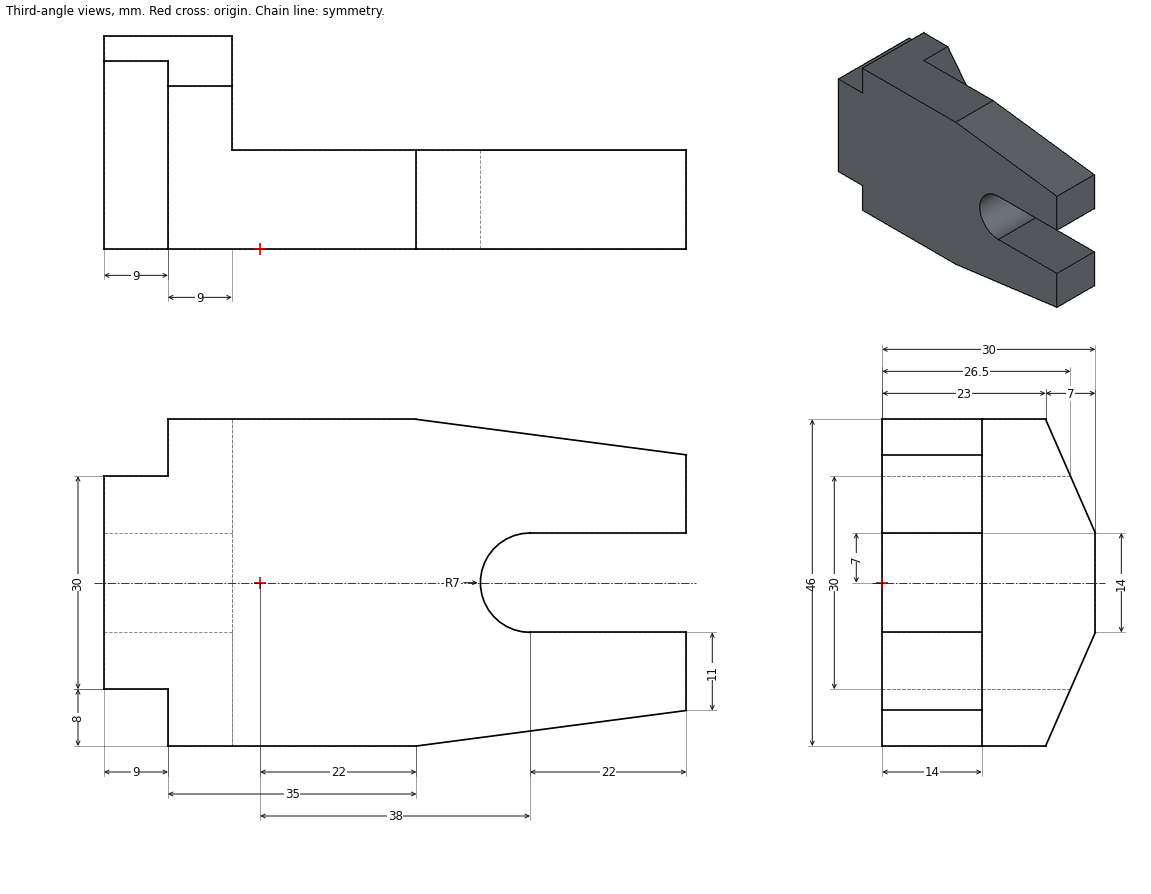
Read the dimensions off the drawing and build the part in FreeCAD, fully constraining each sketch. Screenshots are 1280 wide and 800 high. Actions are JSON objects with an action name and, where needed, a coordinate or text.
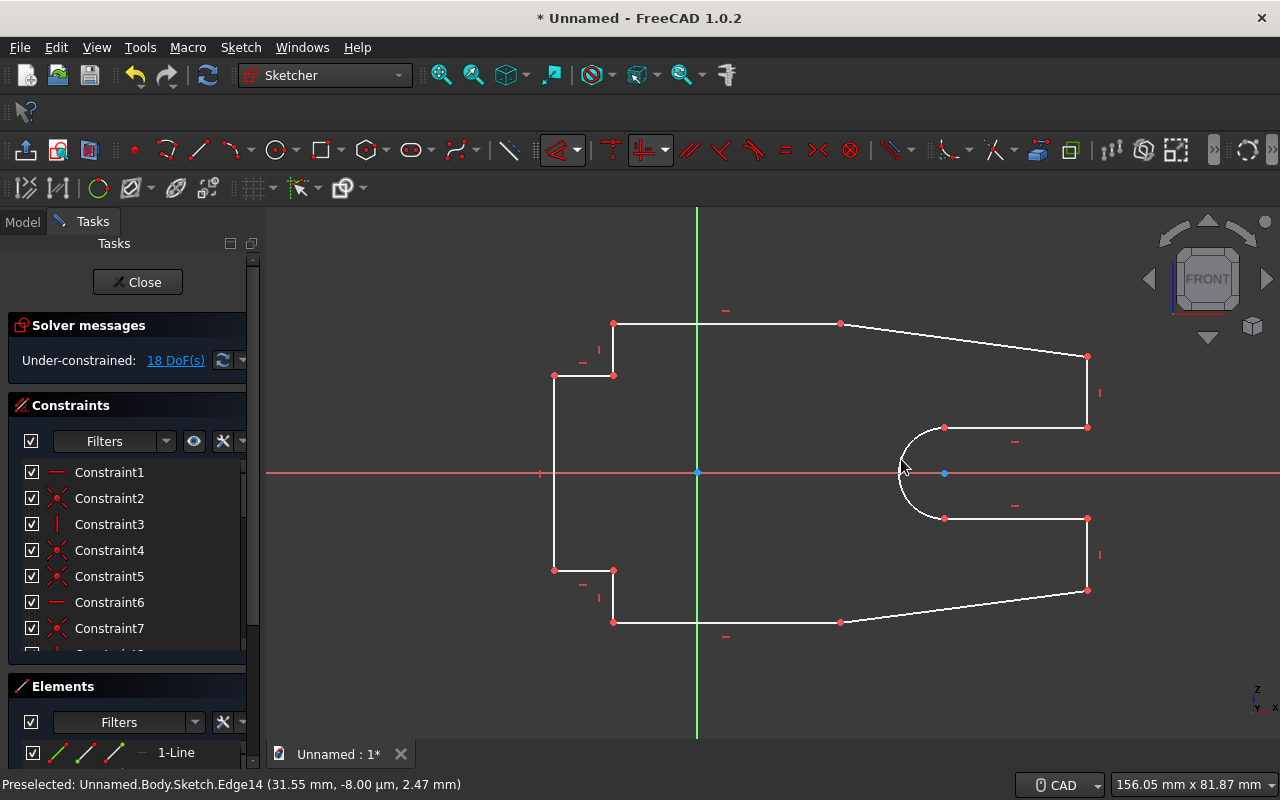
{"action": "left_click", "coordinate": [987, 519]}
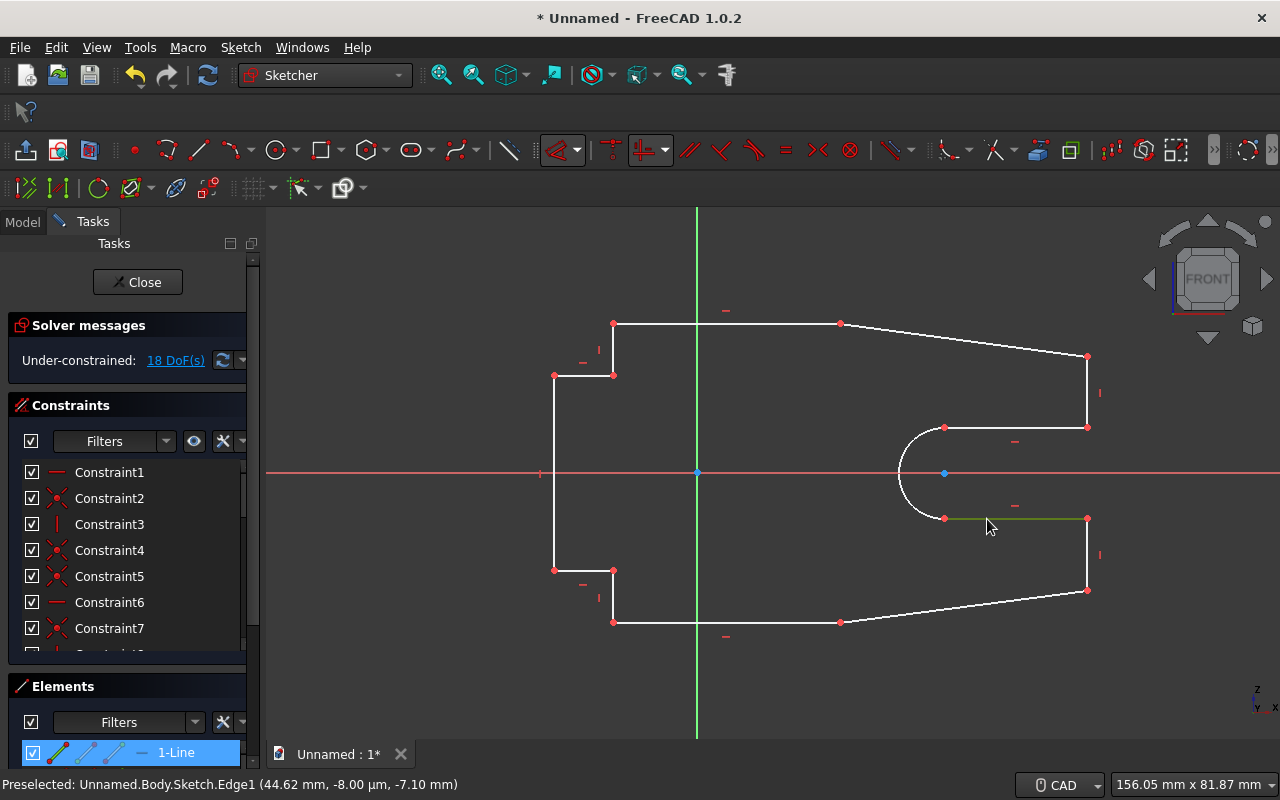
{"action": "left_click", "coordinate": [908, 447]}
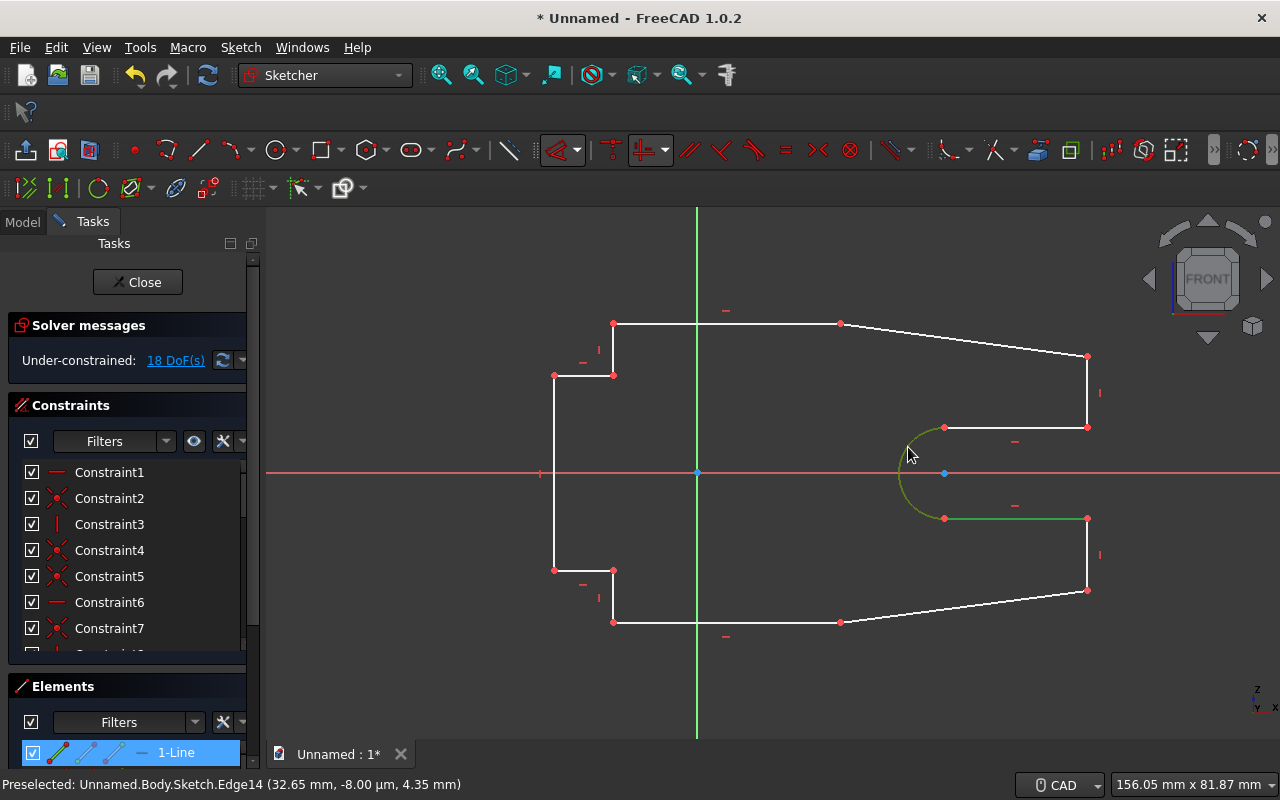
{"action": "left_click", "coordinate": [754, 150]}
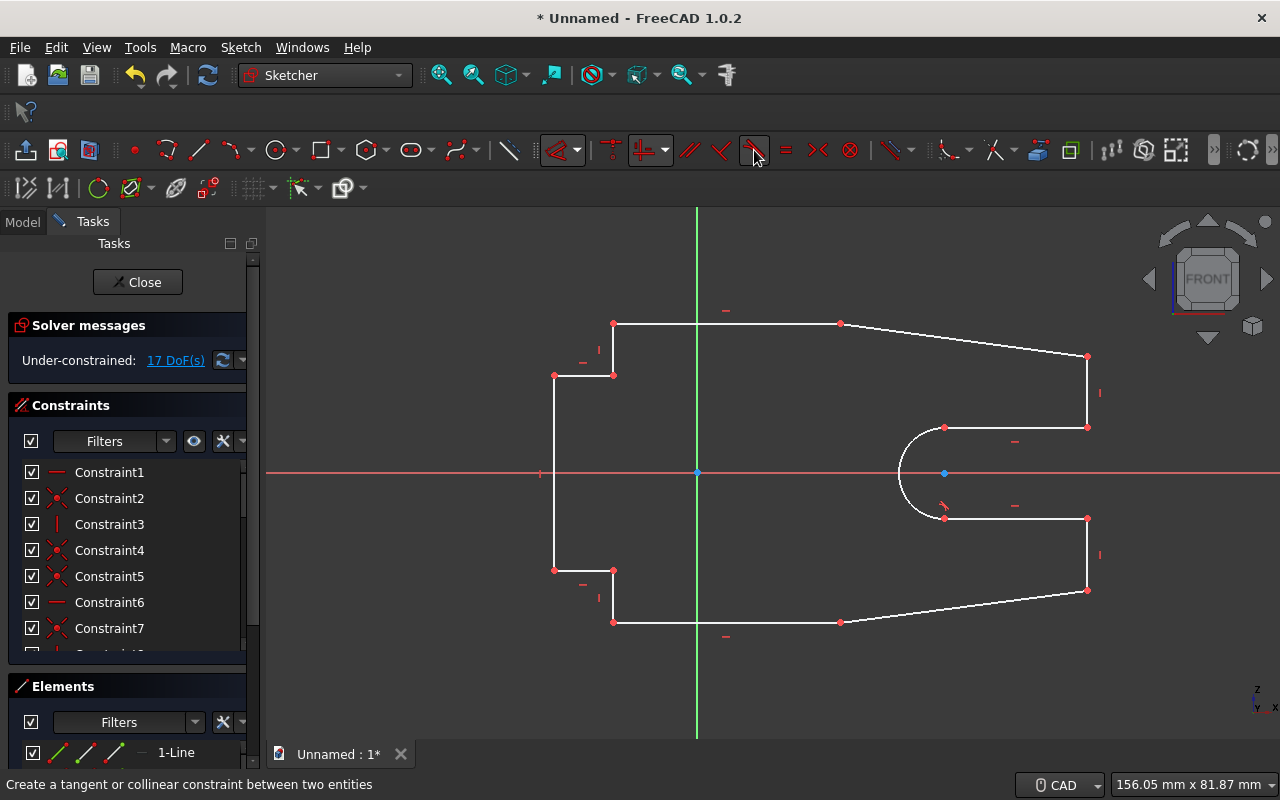
{"action": "left_click", "coordinate": [1044, 428]}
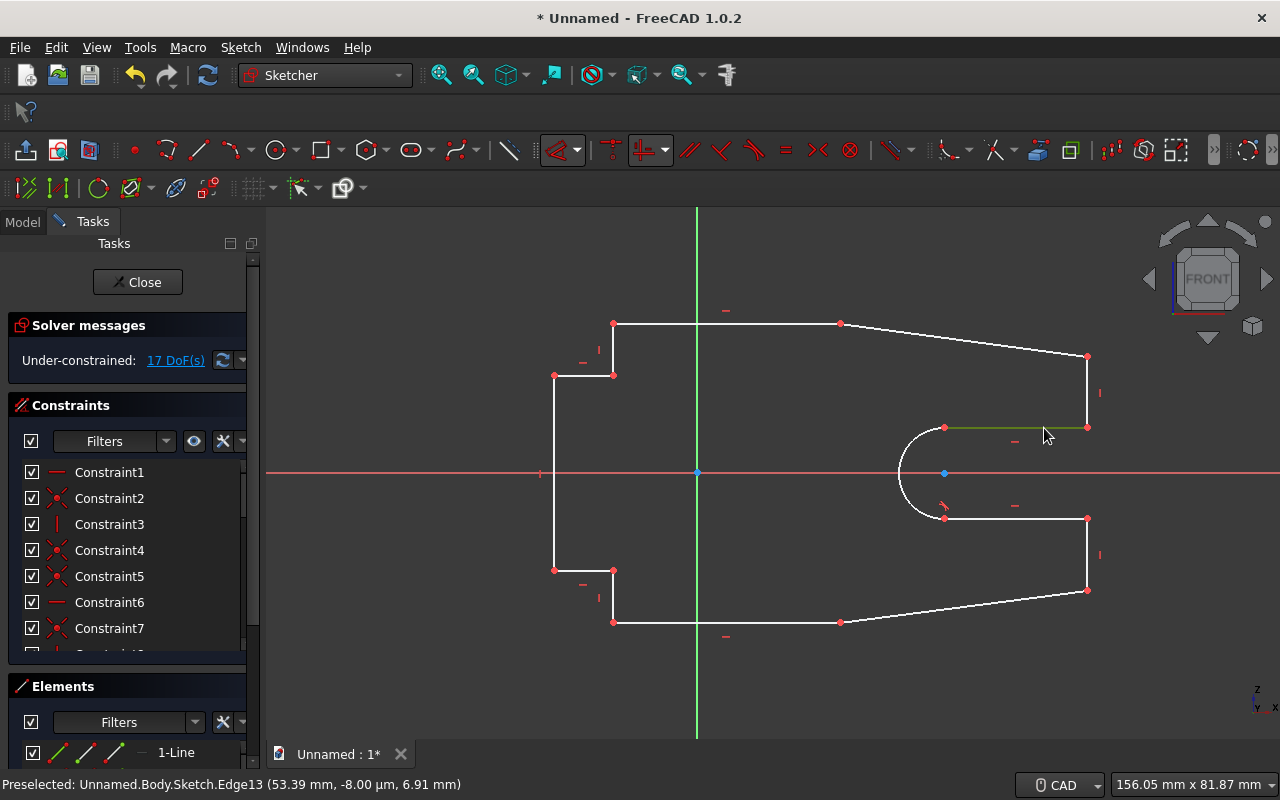
{"action": "left_click", "coordinate": [907, 447]}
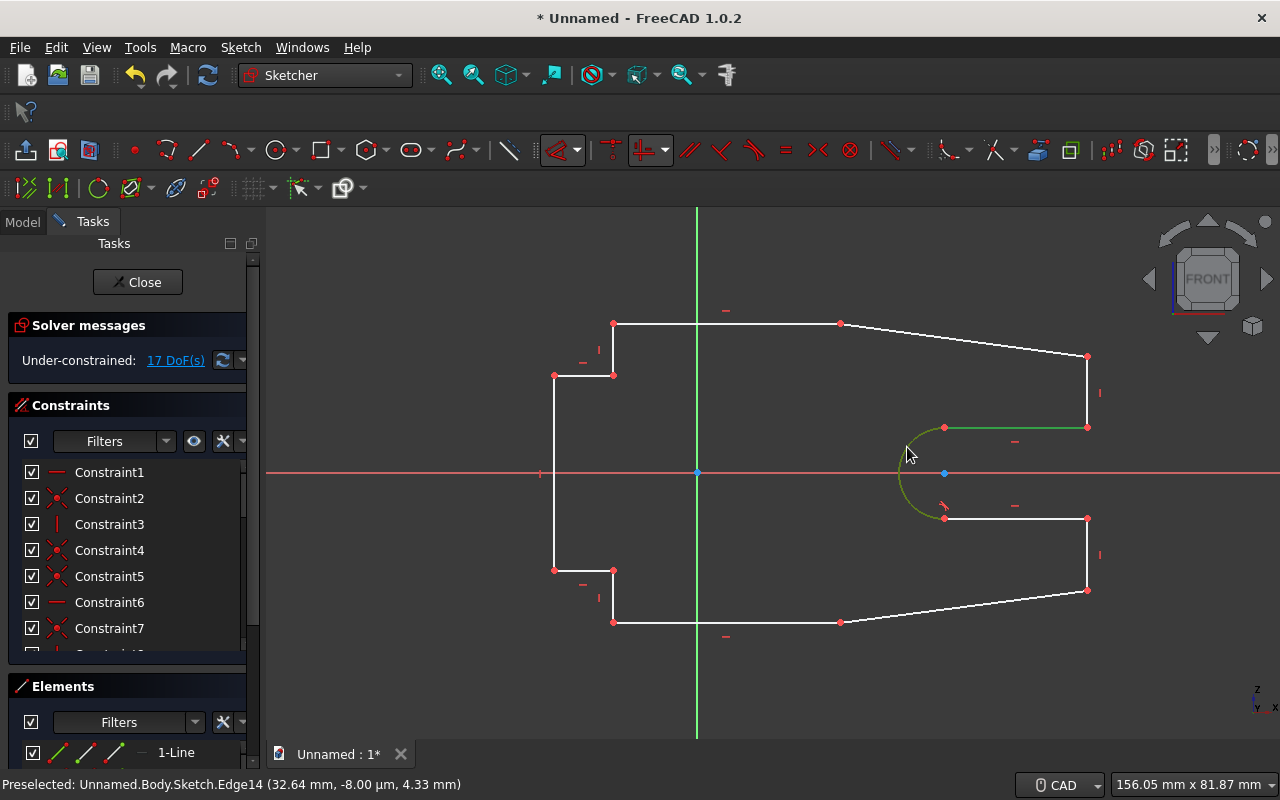
{"action": "key", "text": "t"}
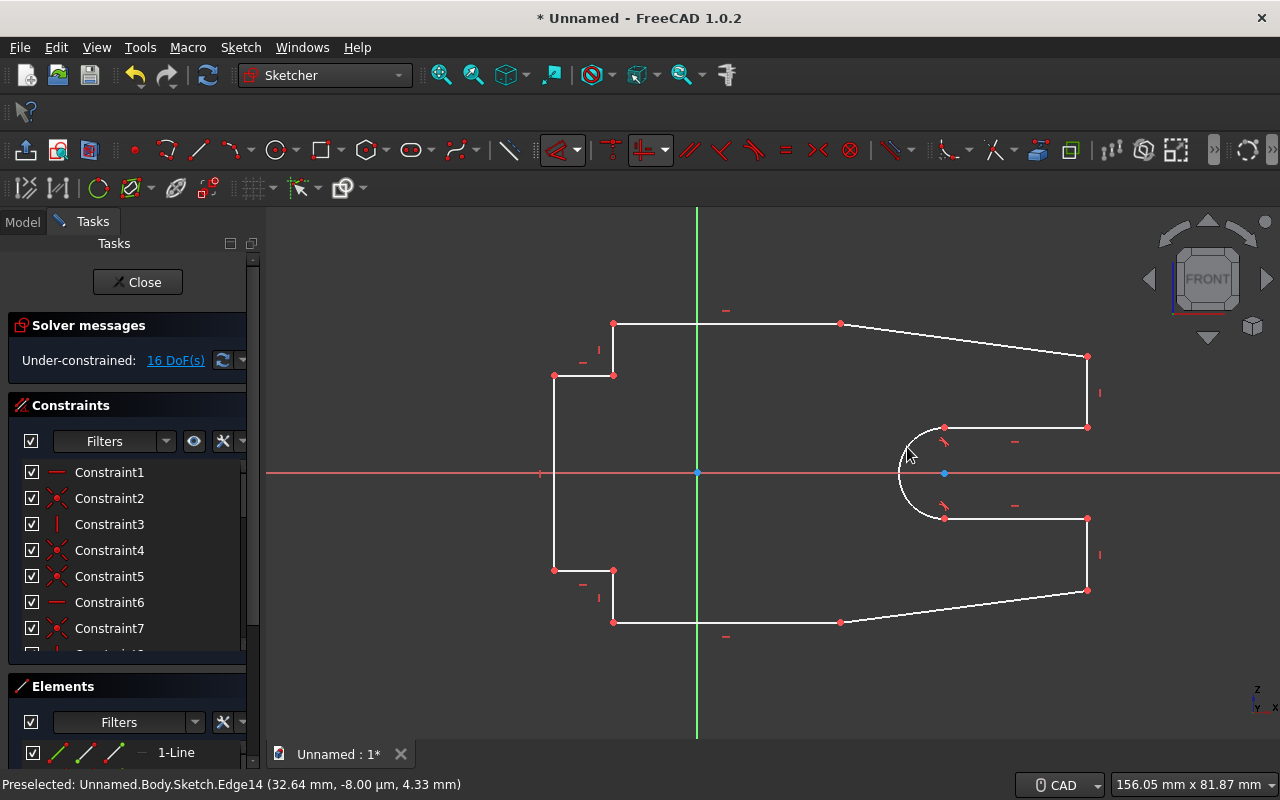
{"action": "left_click", "coordinate": [944, 474]}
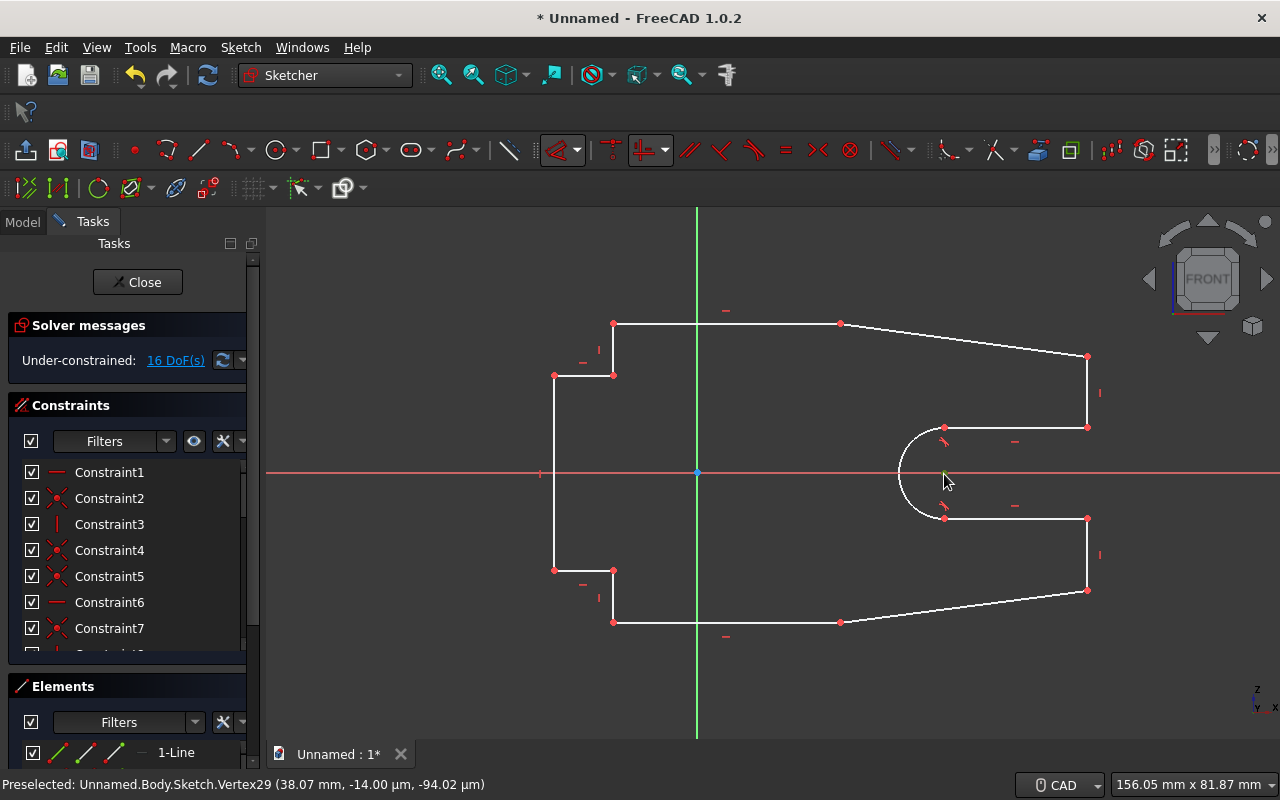
{"action": "left_click", "coordinate": [353, 473]}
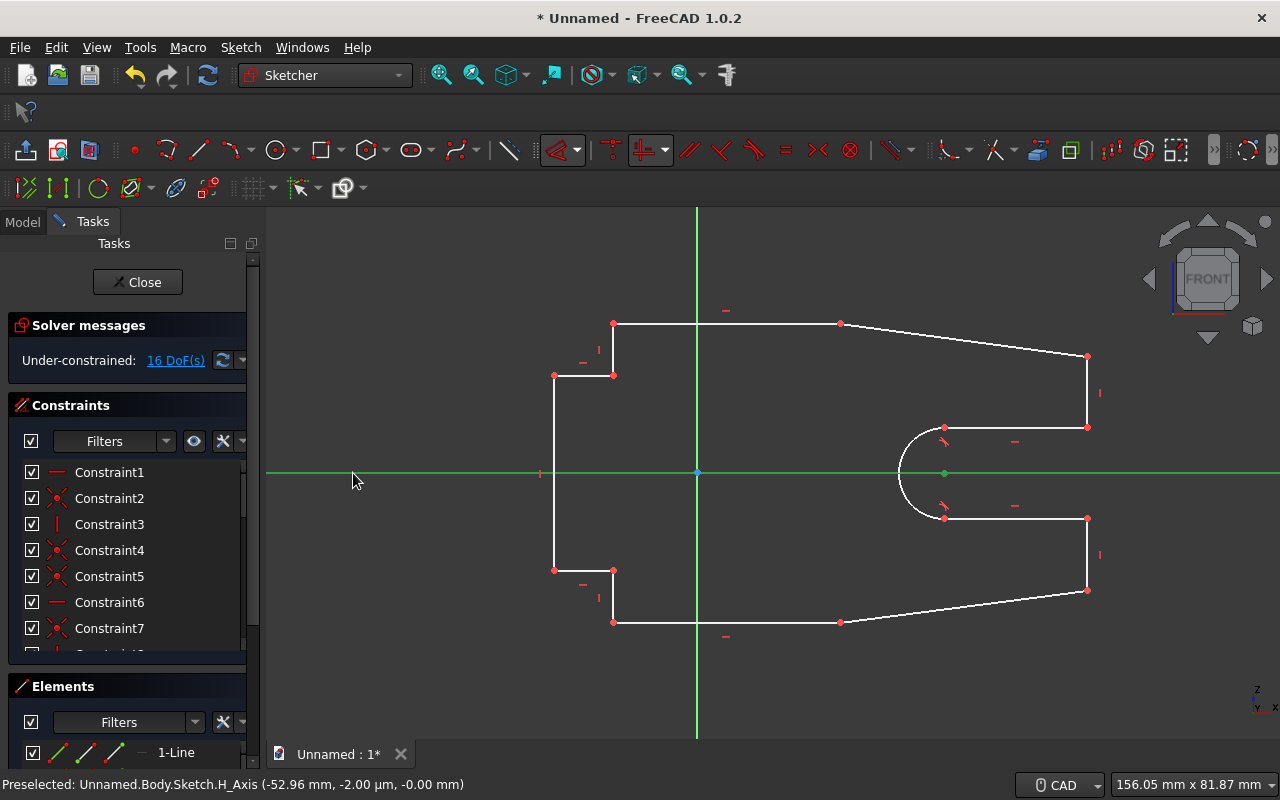
{"action": "key", "text": "c"}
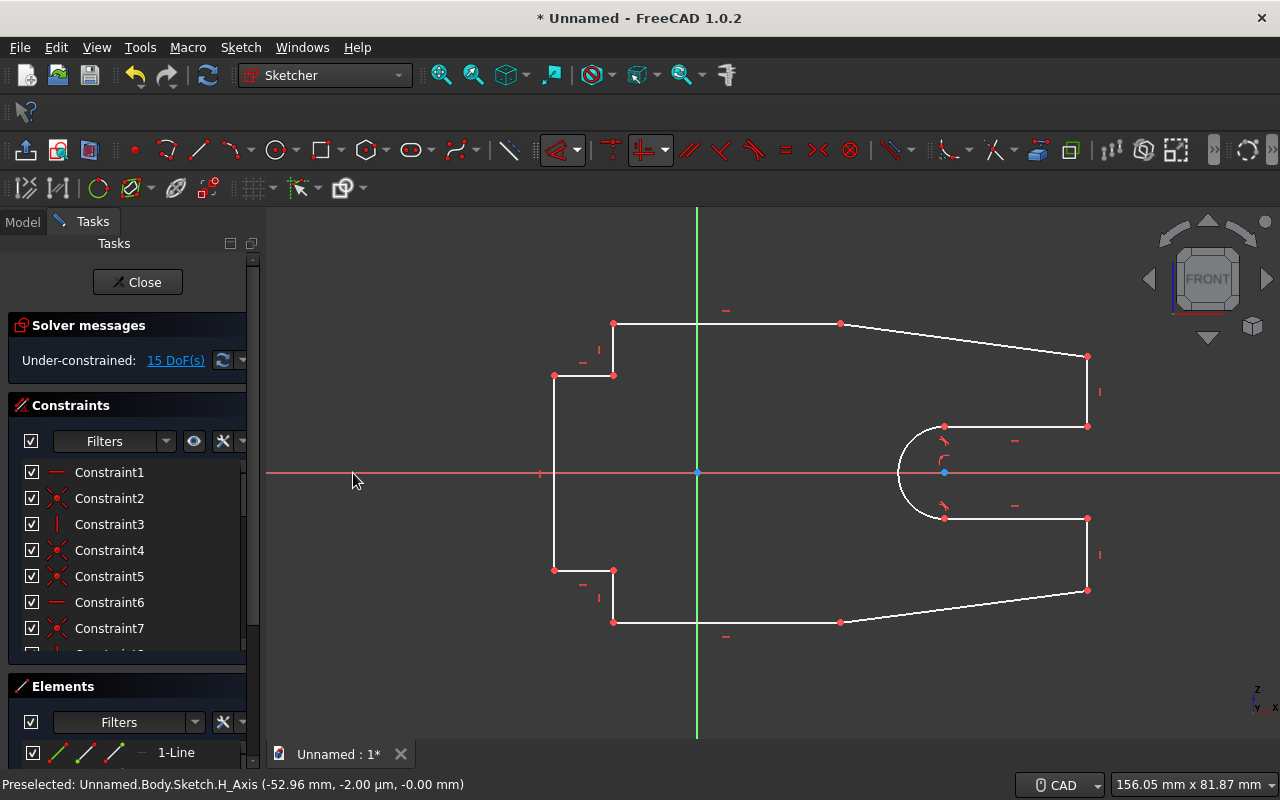
{"action": "left_click", "coordinate": [613, 571]}